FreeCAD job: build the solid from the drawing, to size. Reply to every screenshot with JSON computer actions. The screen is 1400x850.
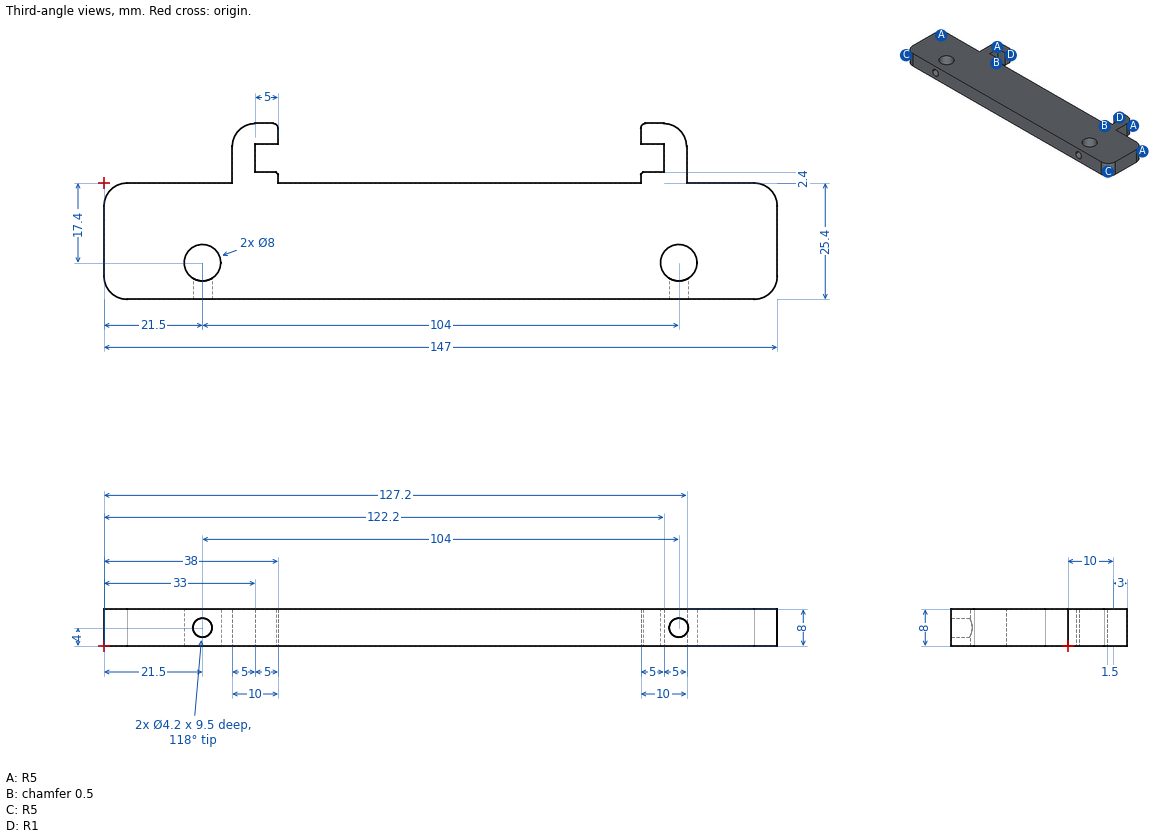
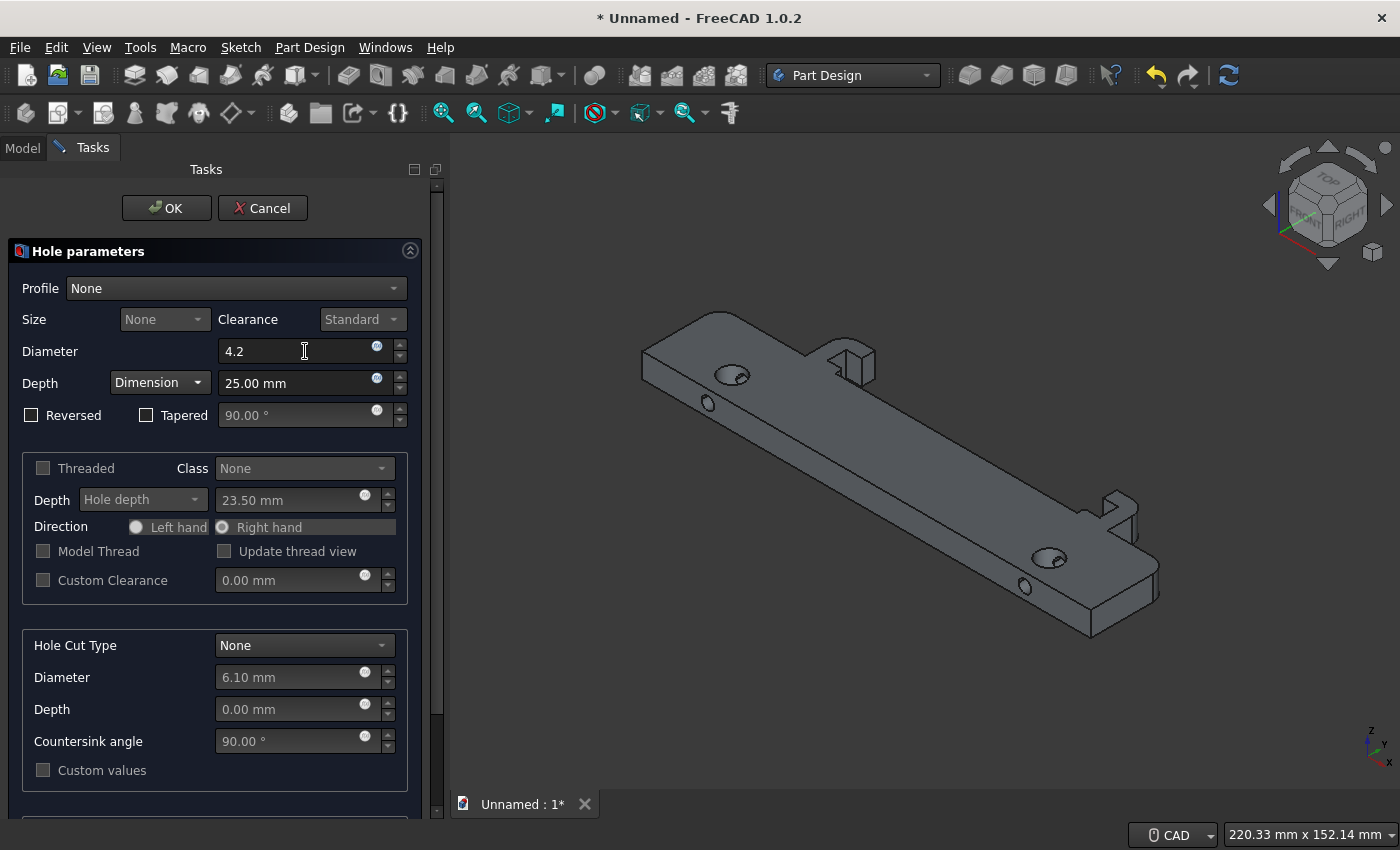
{"action": "triple_click", "coordinate": [305, 383]}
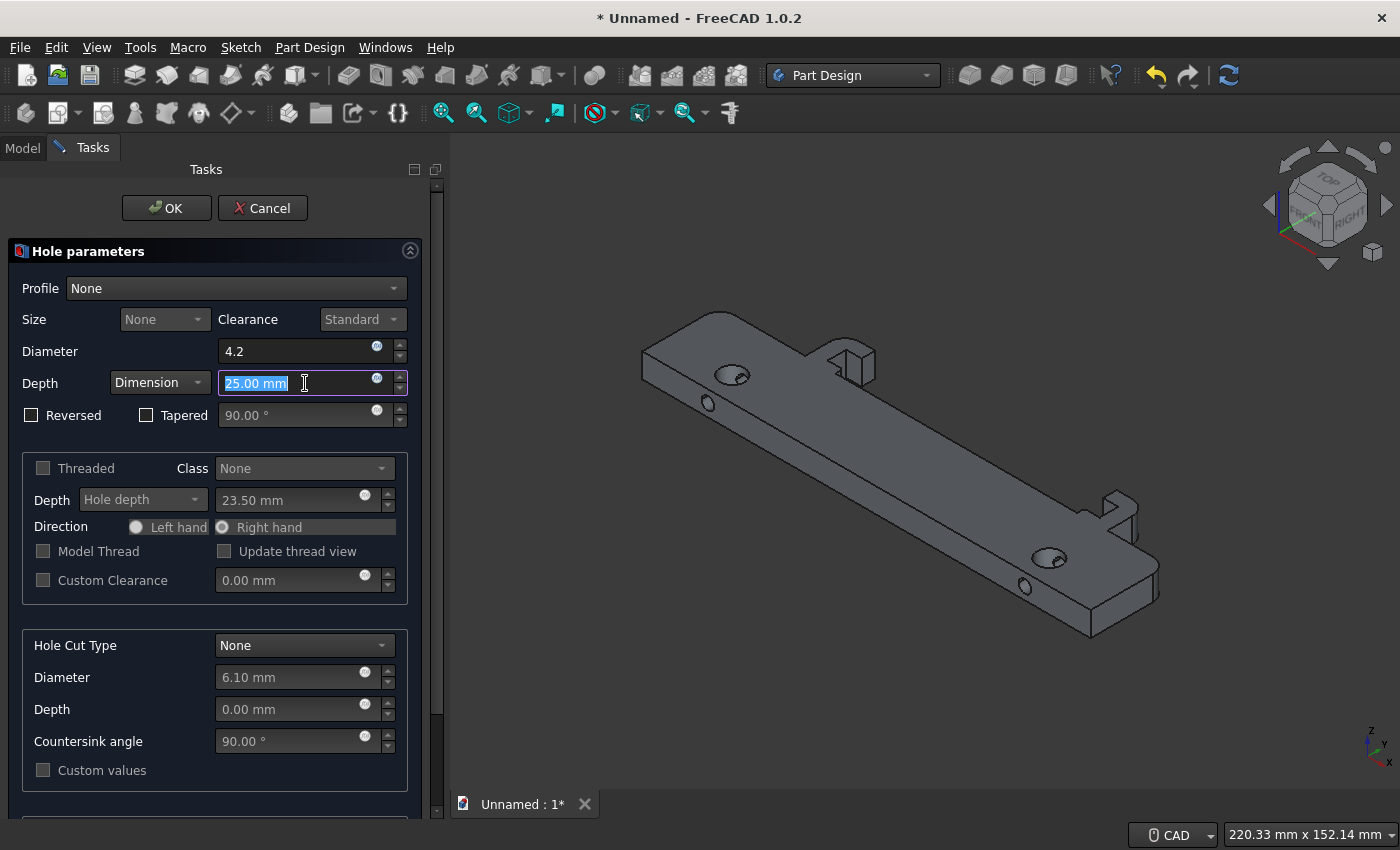
{"action": "type", "text": "9.5"}
{"action": "key", "text": "Tab"}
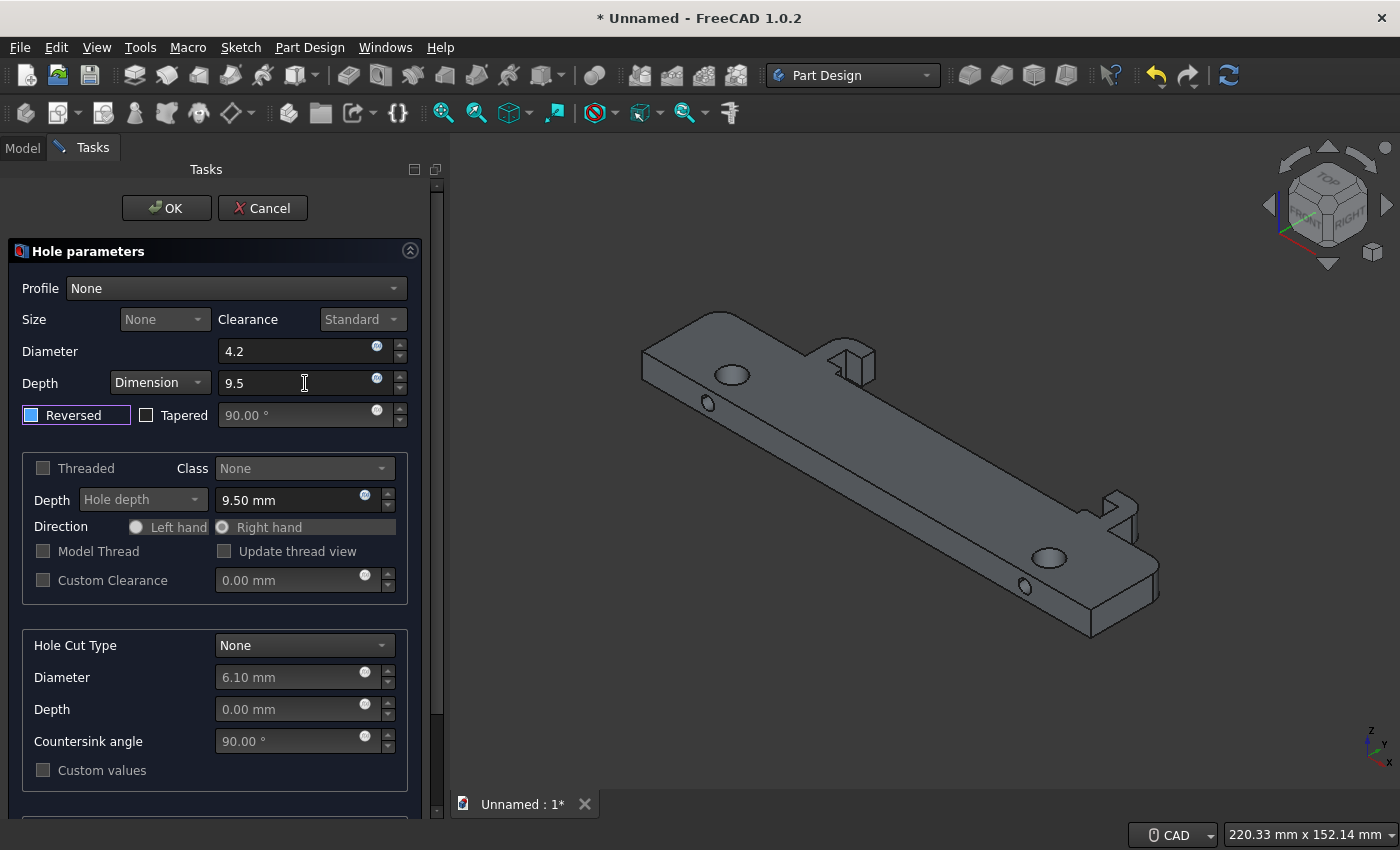
{"action": "left_click", "coordinate": [167, 208]}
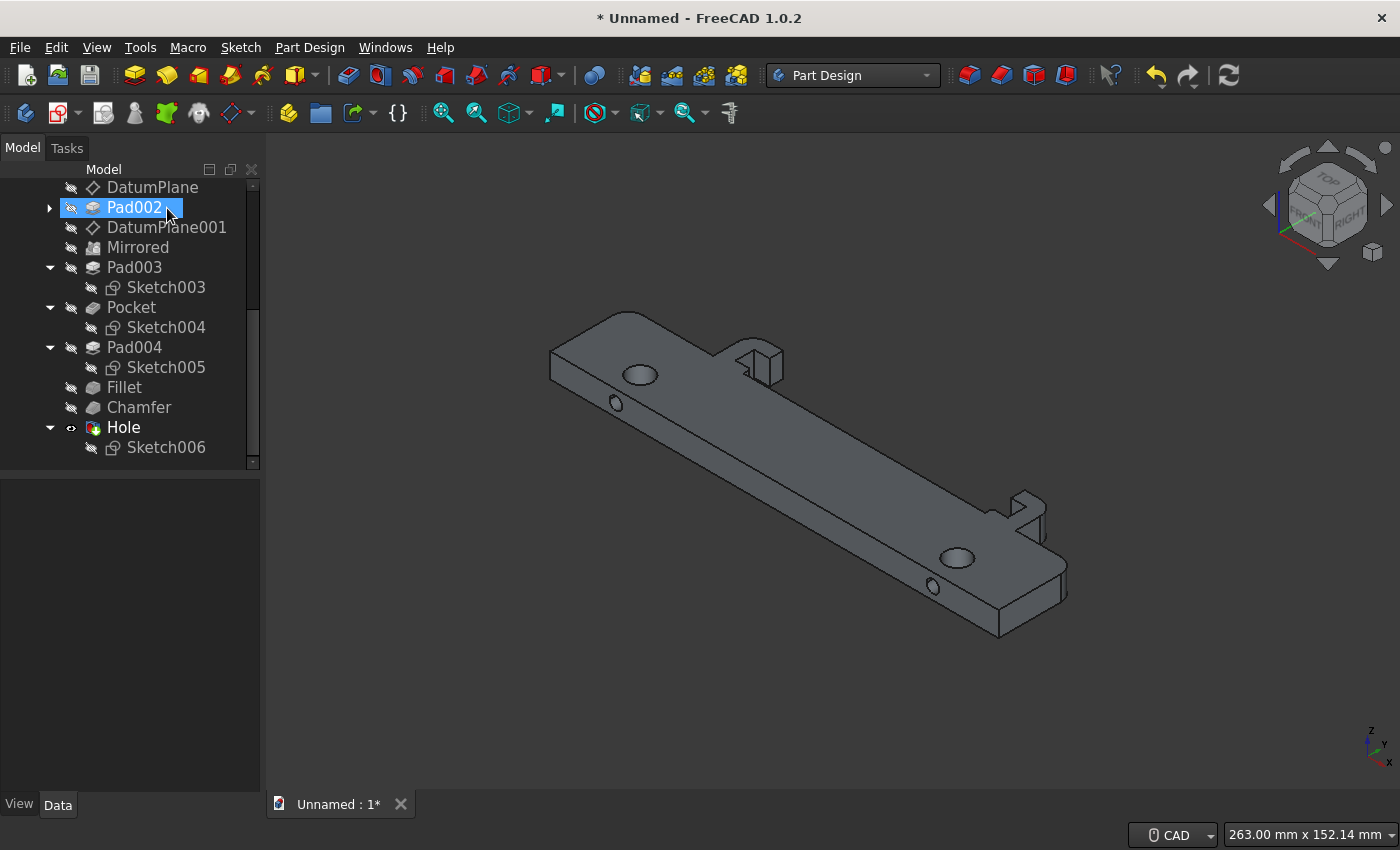
{"action": "left_click", "coordinate": [999, 623]}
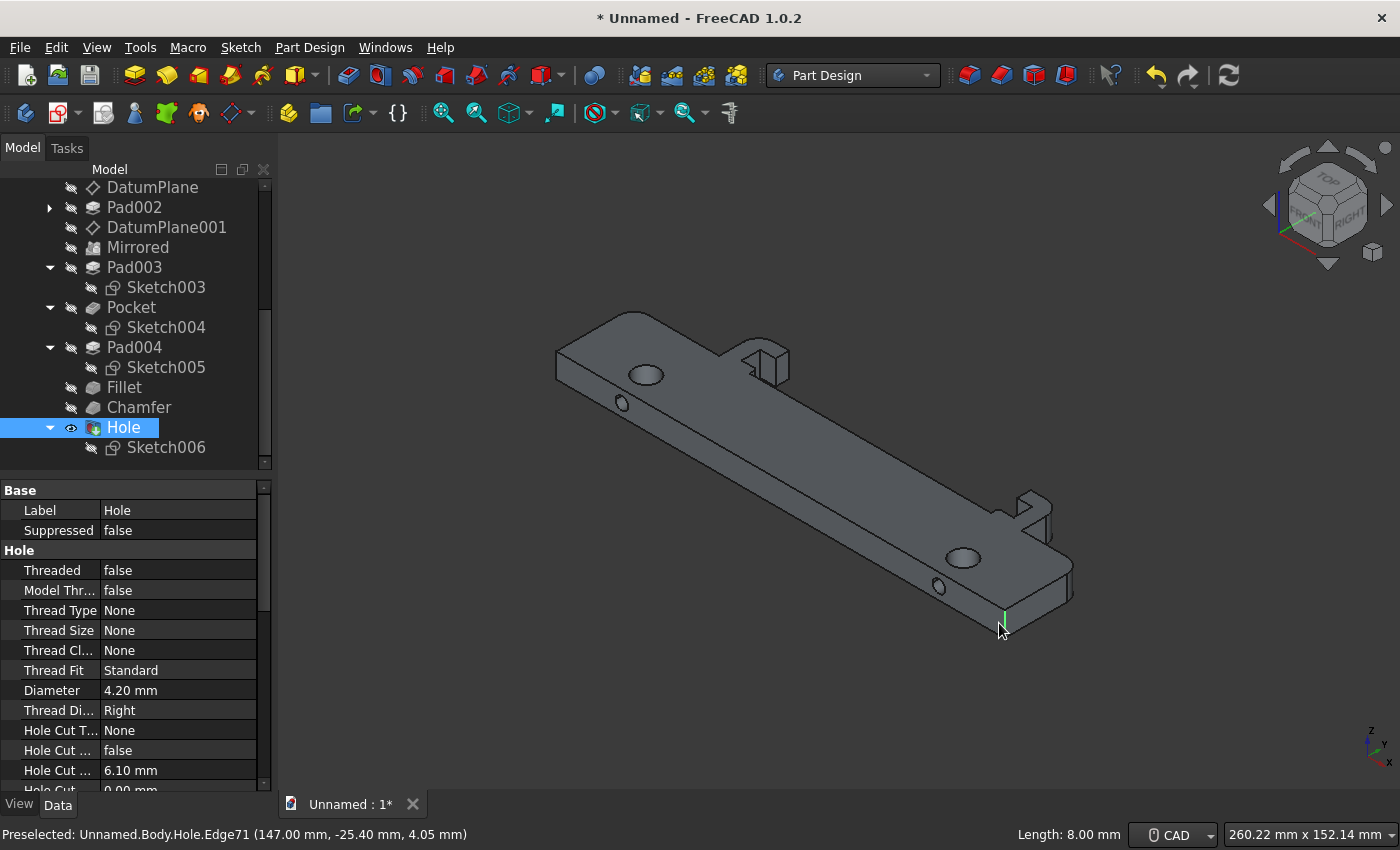
{"action": "key", "text": "2"}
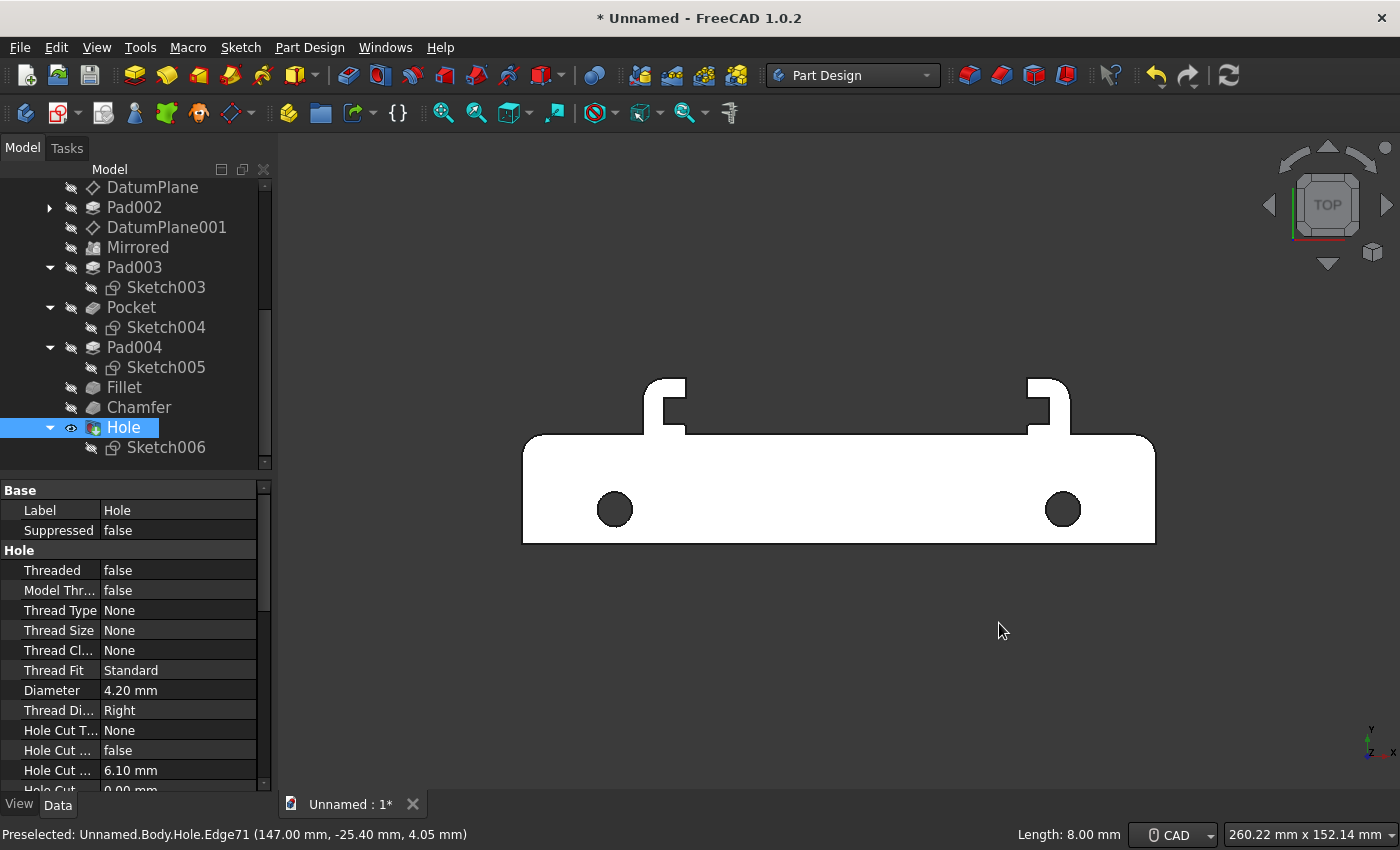
{"action": "key", "text": "0"}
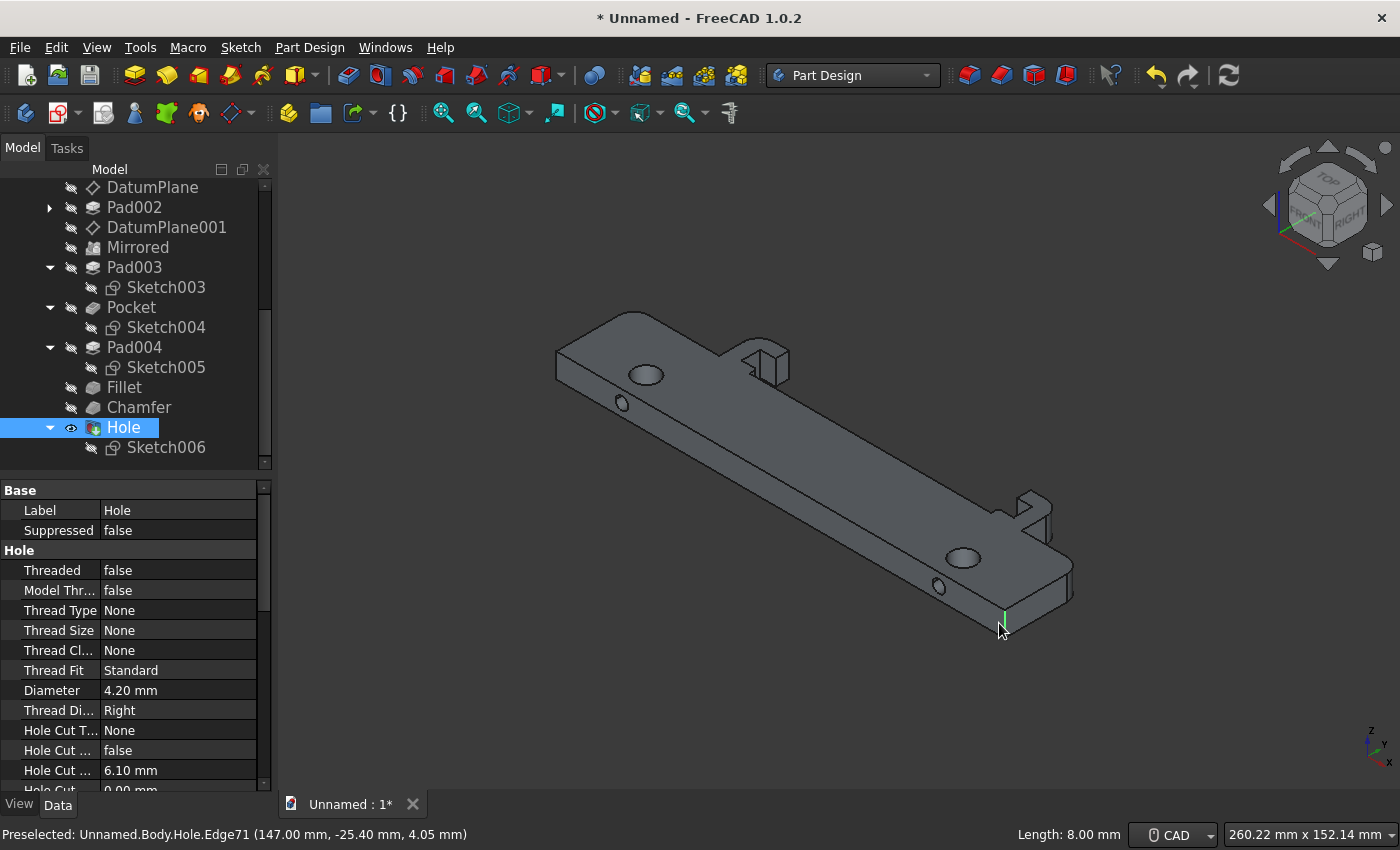
{"action": "key", "text": "1"}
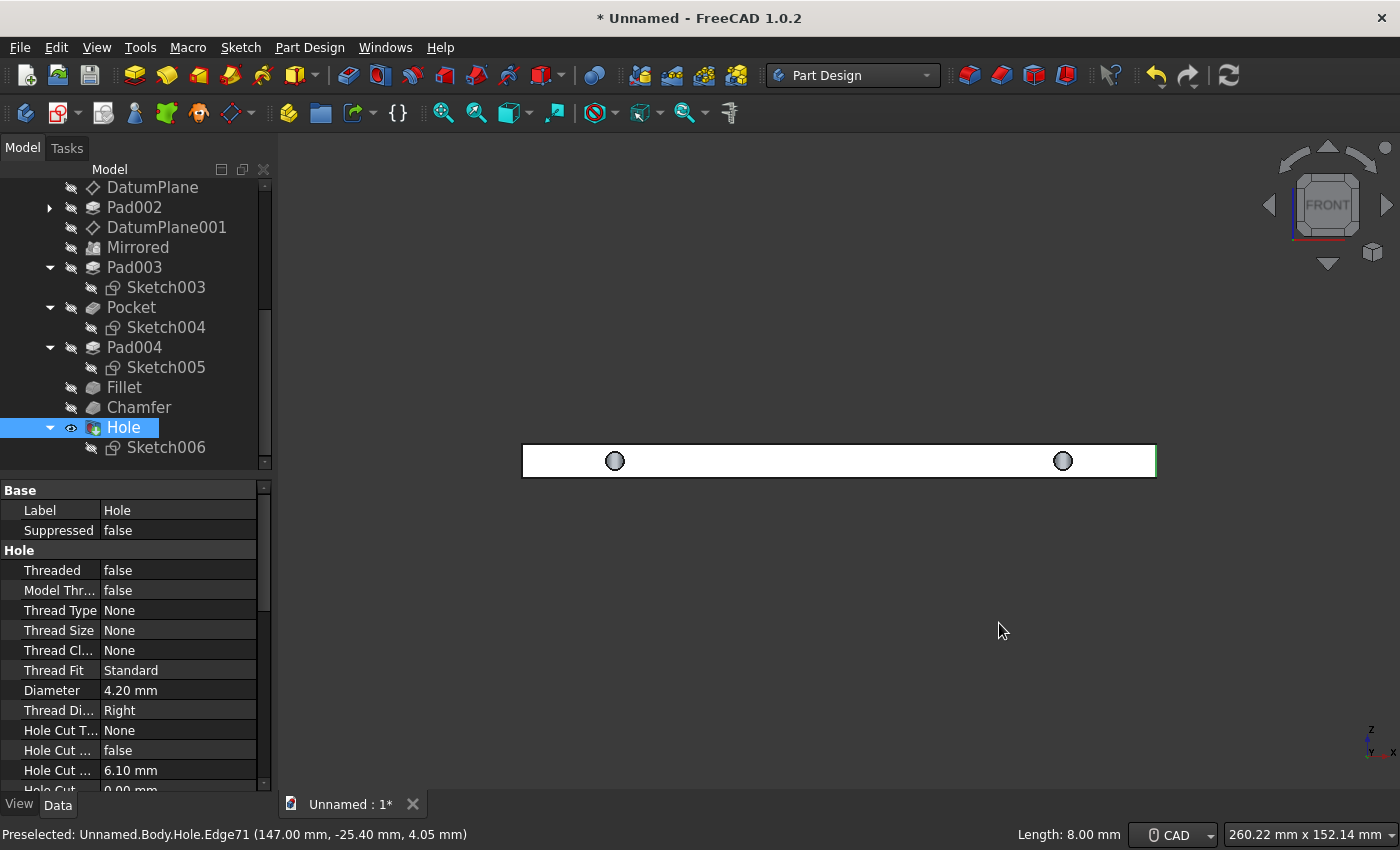
{"action": "left_click", "coordinate": [522, 460], "text": "ctrl"}